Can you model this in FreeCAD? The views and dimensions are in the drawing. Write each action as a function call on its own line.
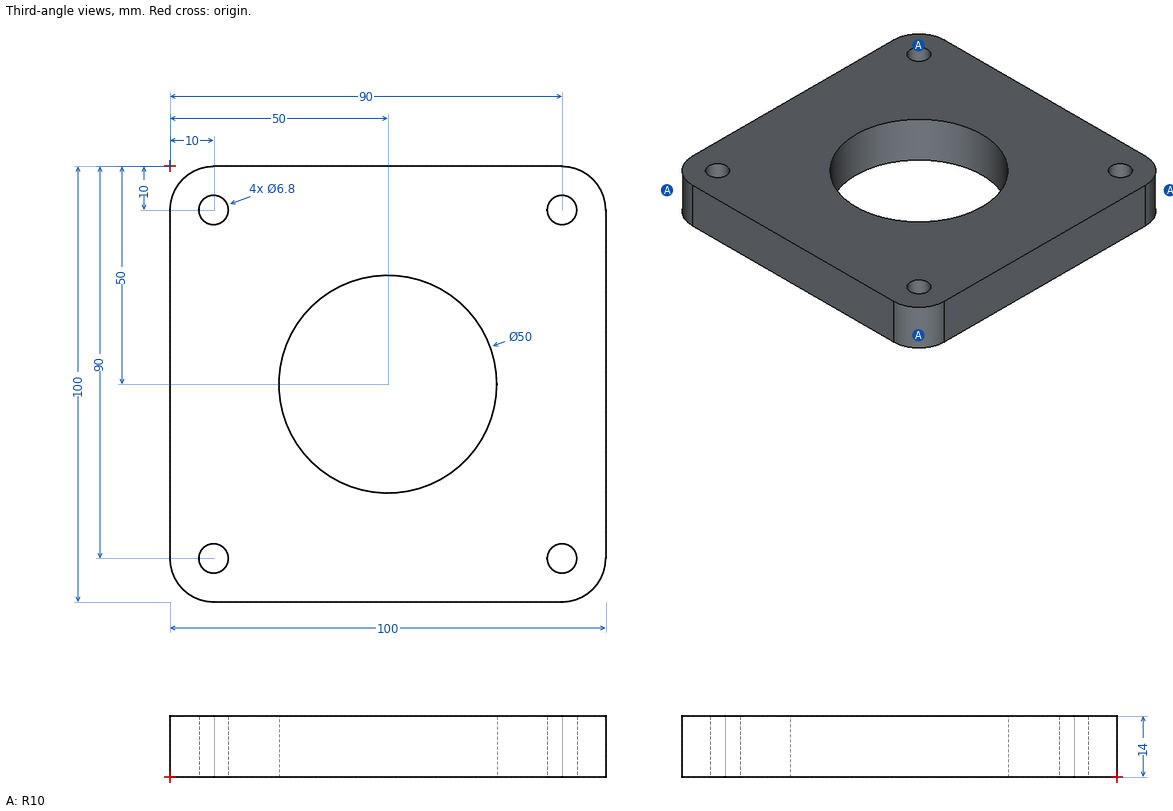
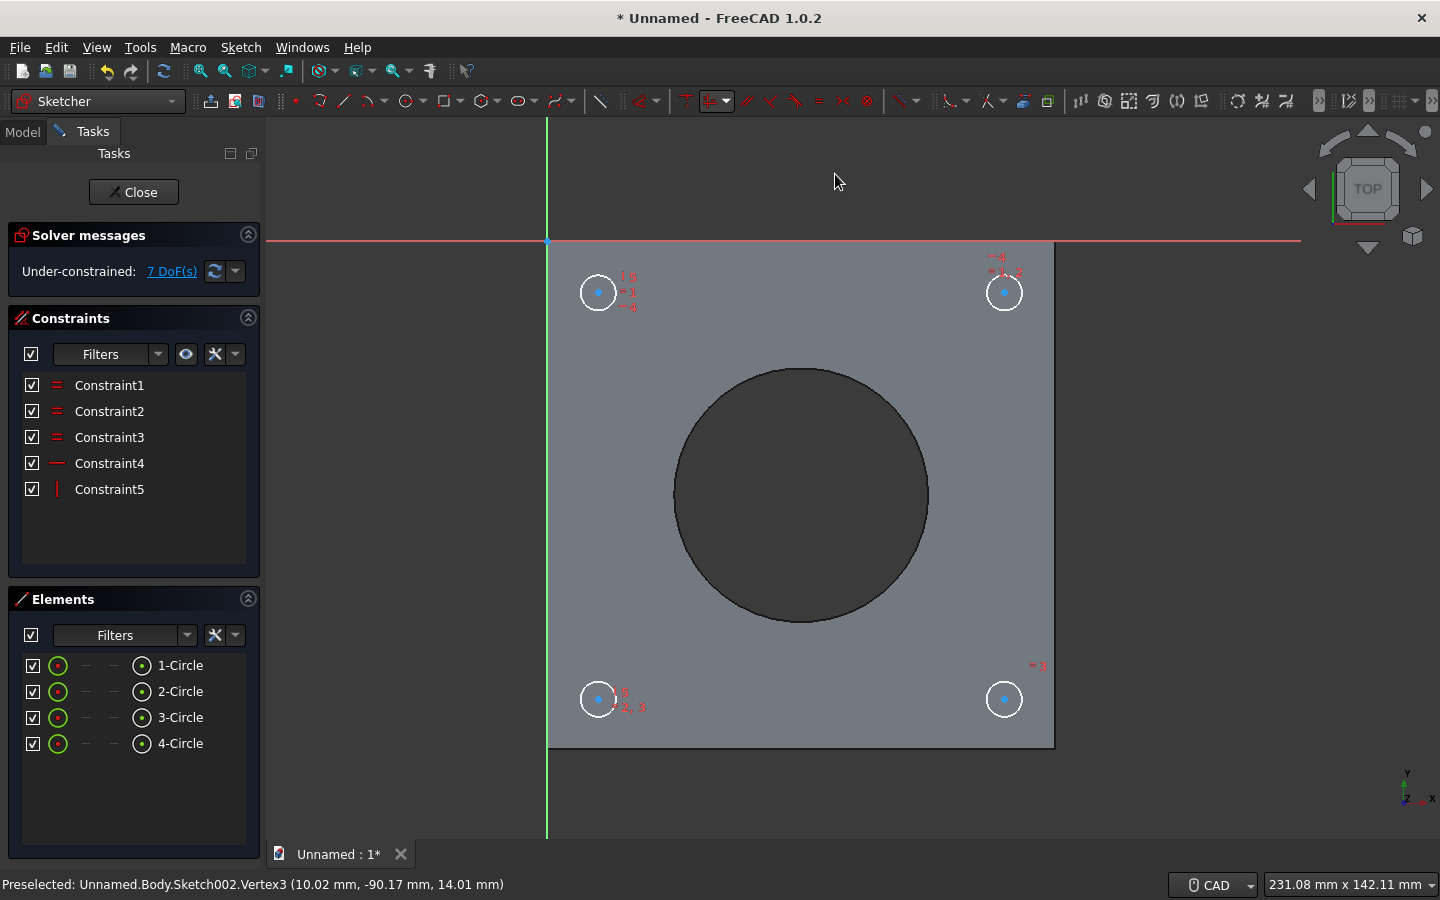
click(1005, 293)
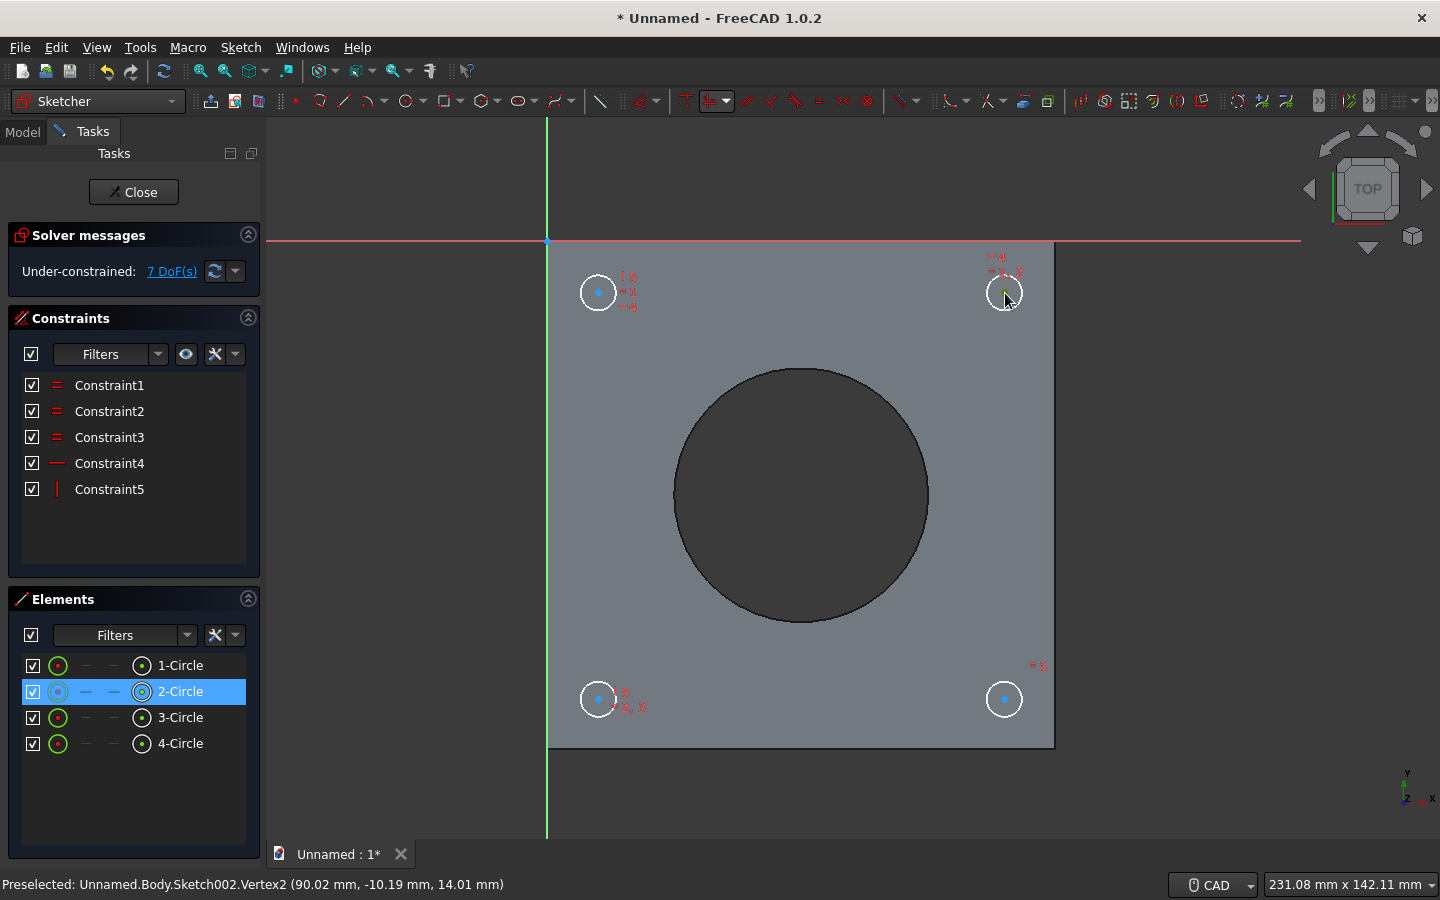
click(1004, 699)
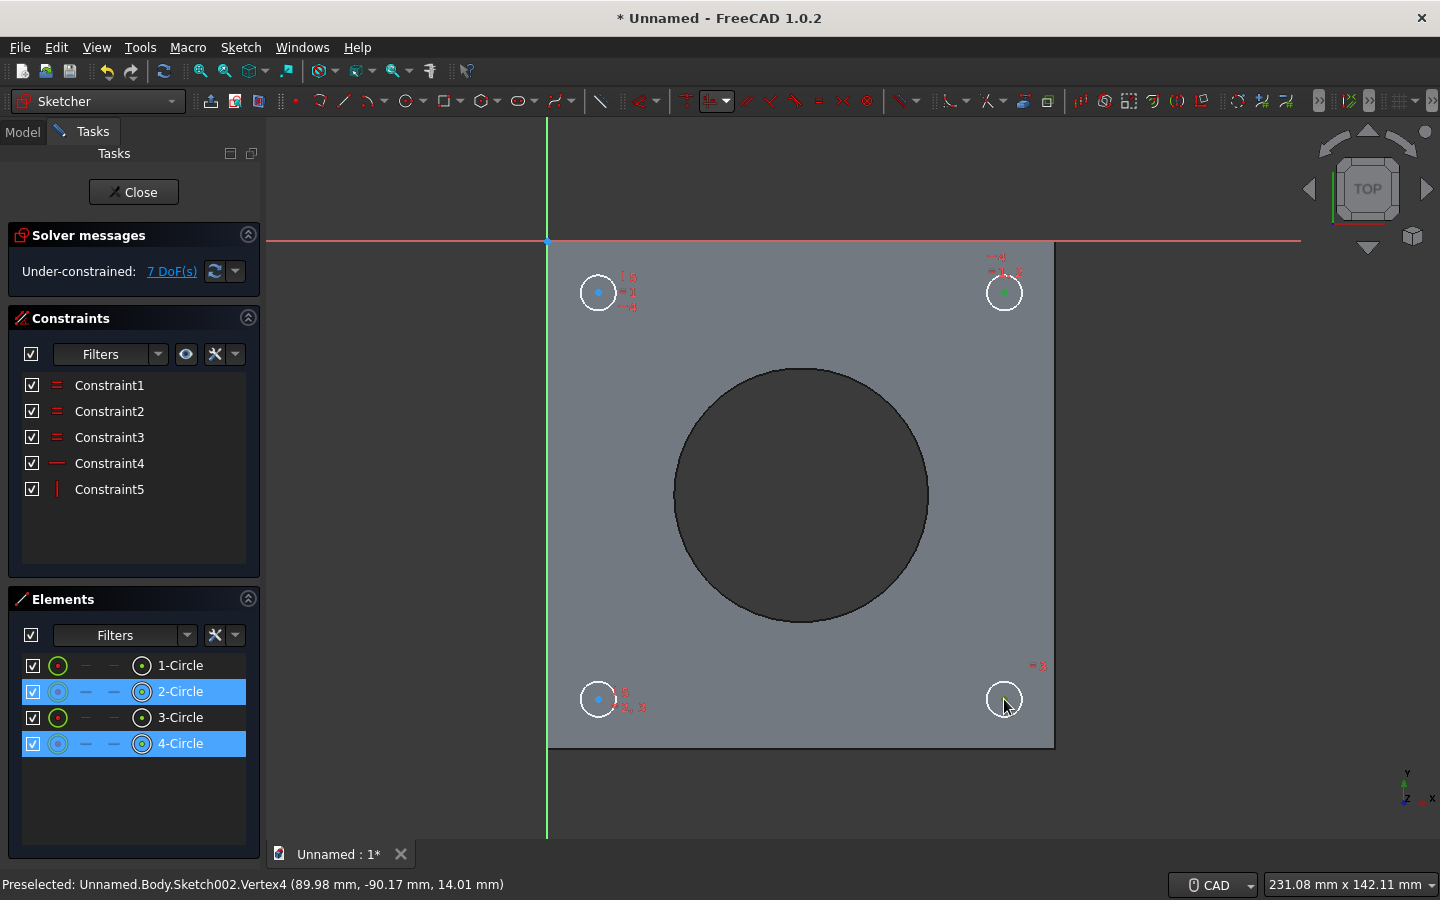
click(728, 102)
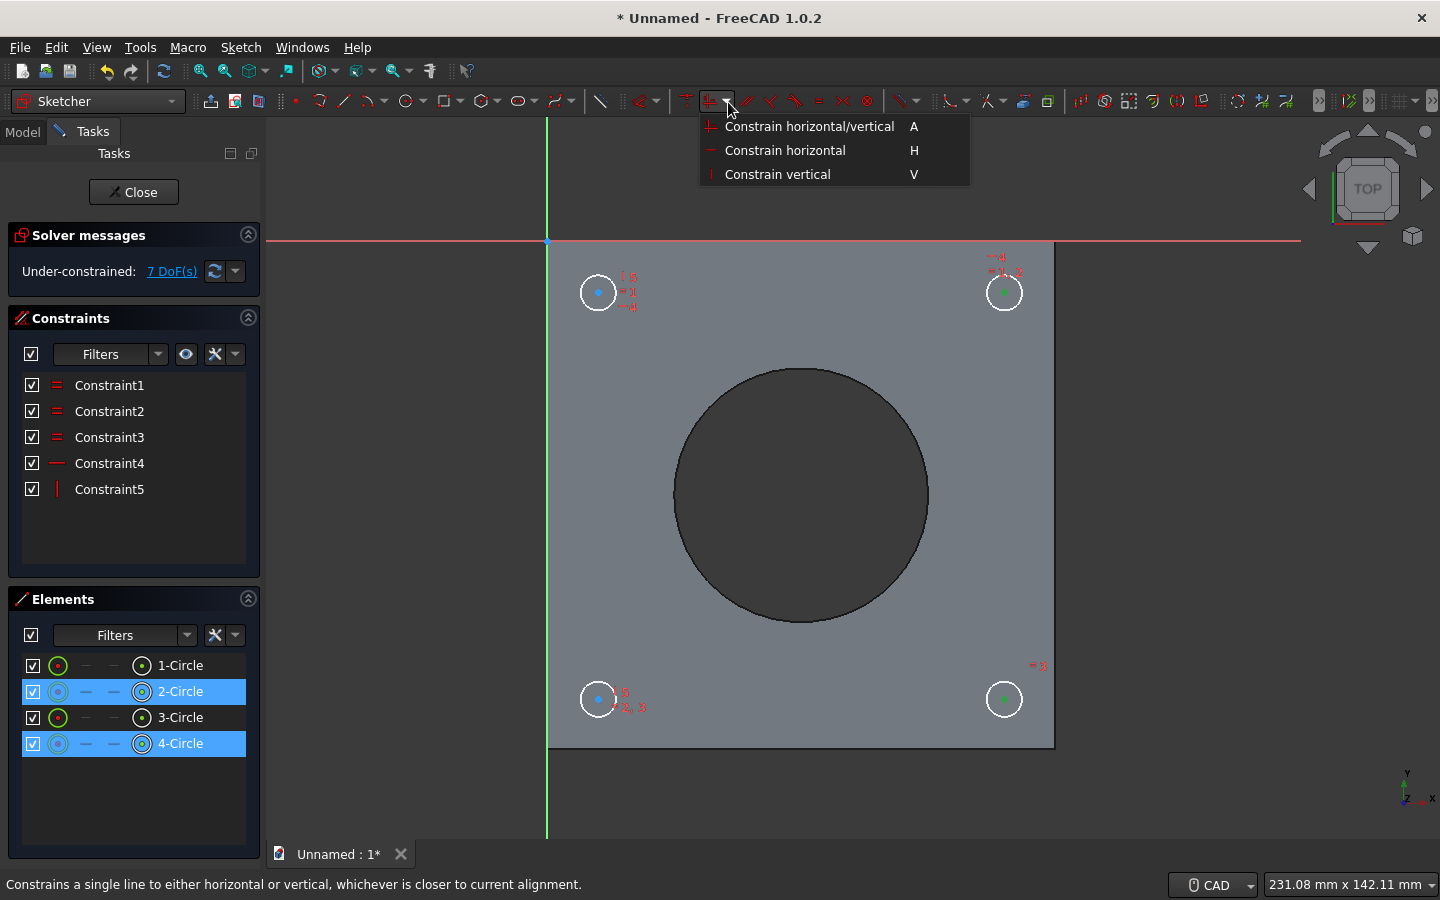
click(835, 174)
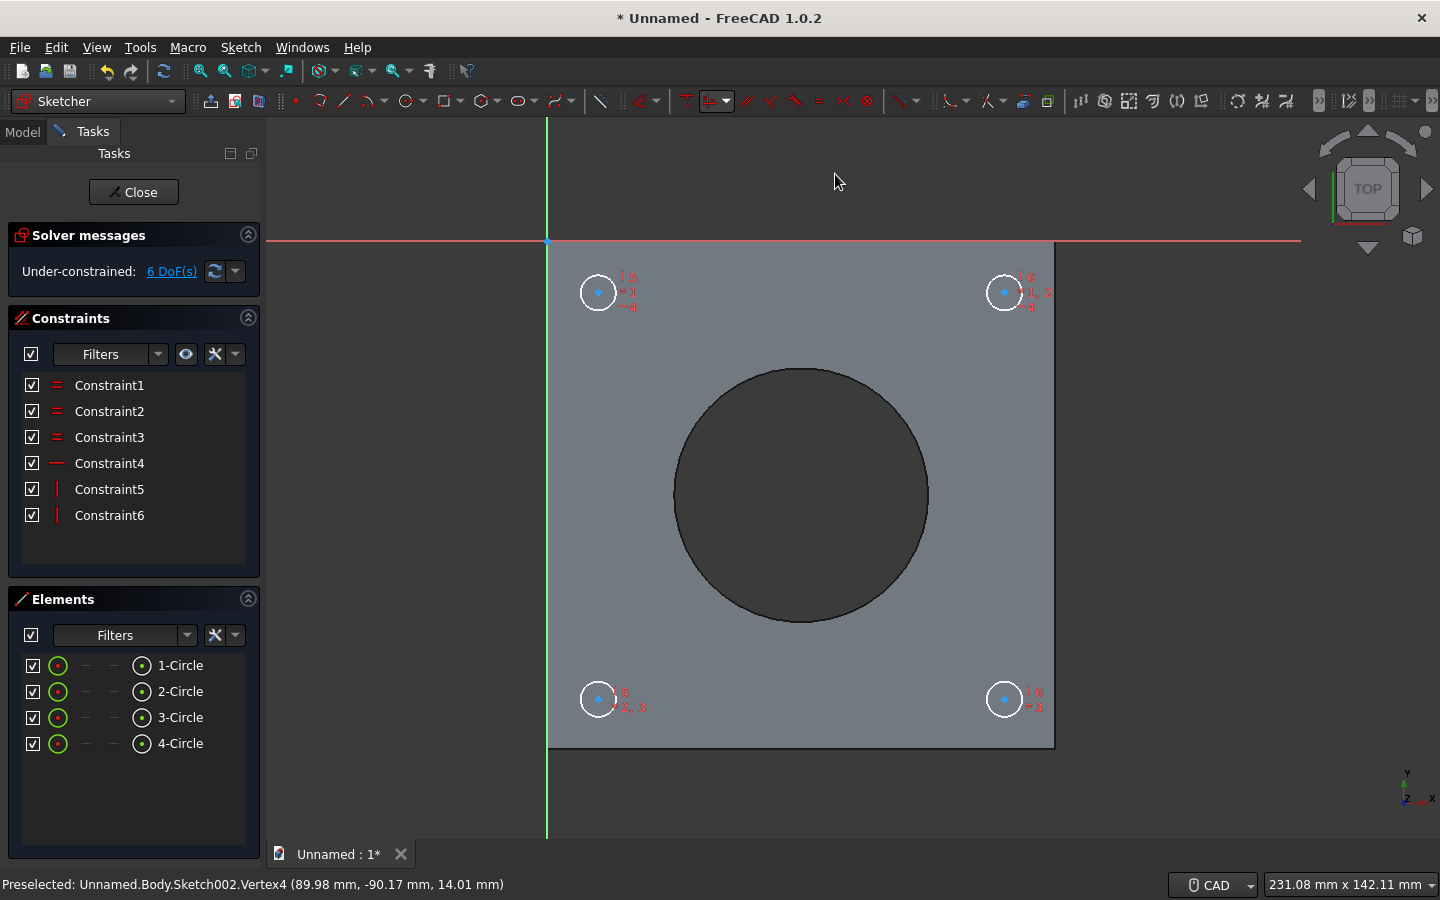
click(598, 699)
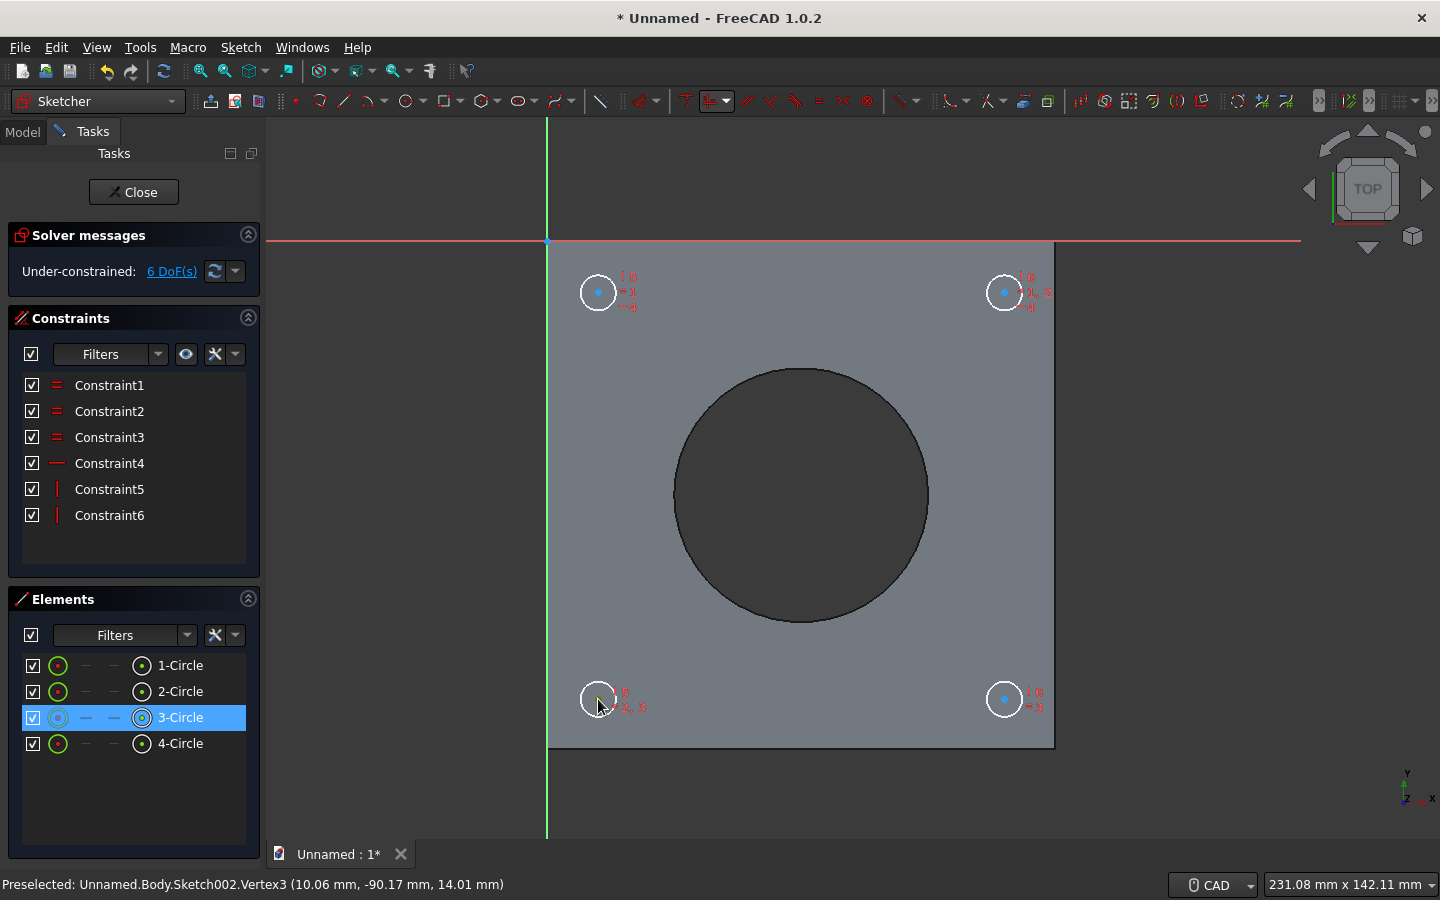
click(1005, 699)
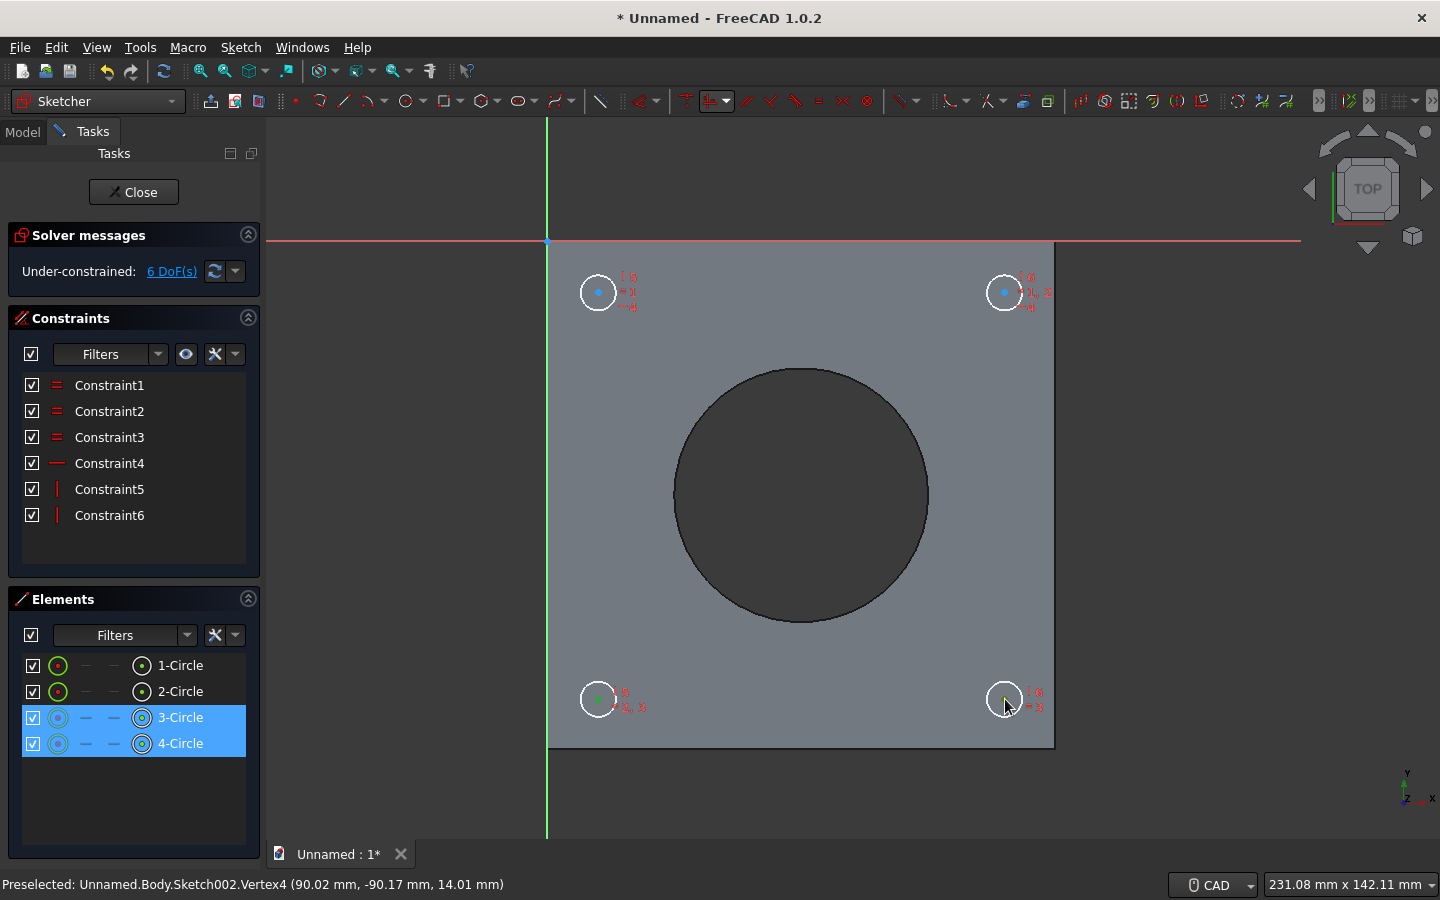
key(h)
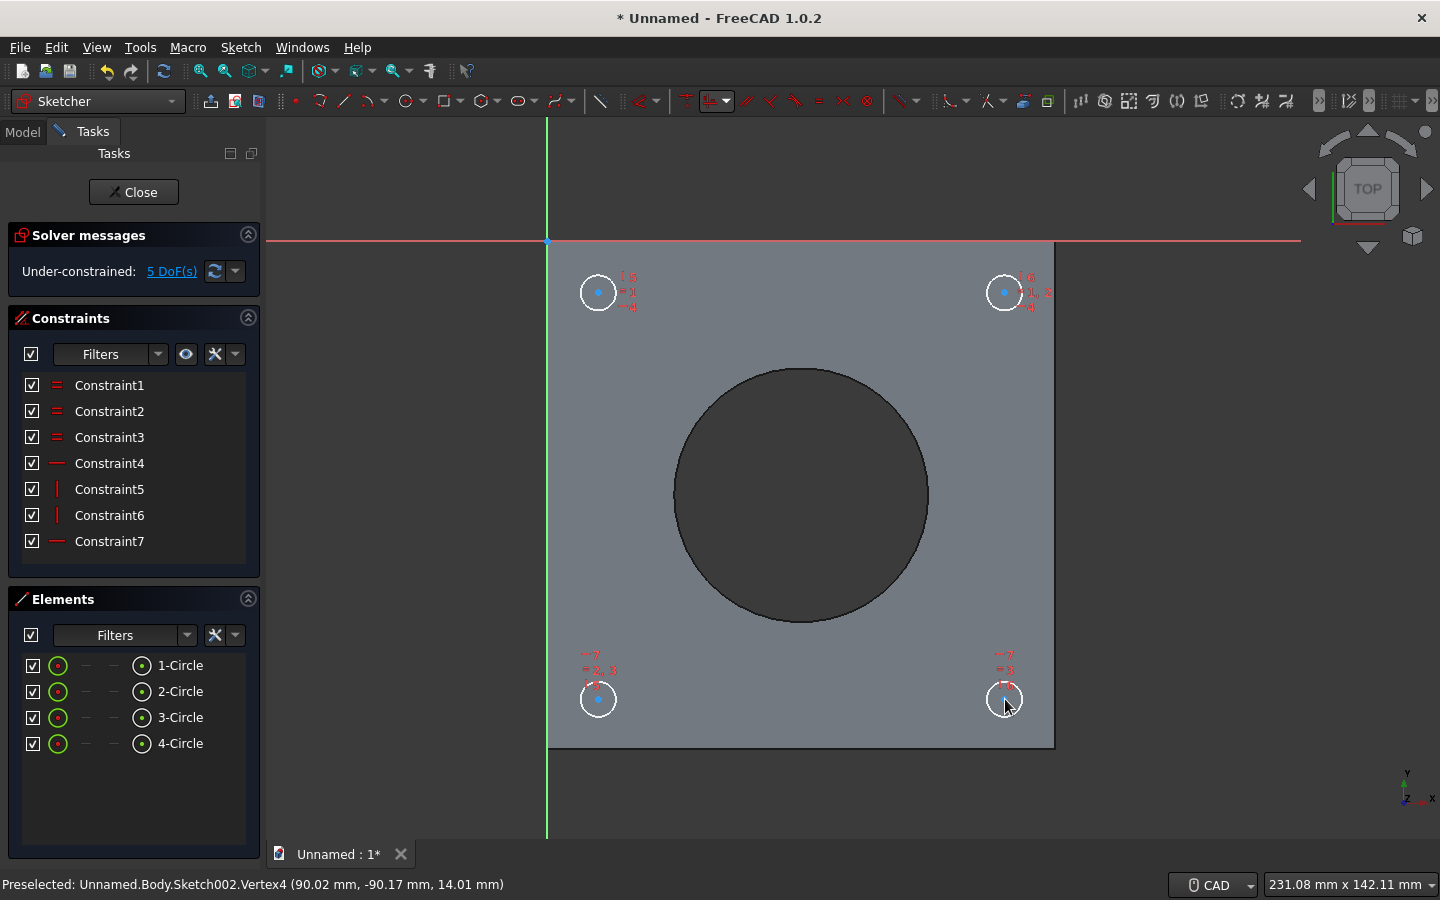
click(640, 102)